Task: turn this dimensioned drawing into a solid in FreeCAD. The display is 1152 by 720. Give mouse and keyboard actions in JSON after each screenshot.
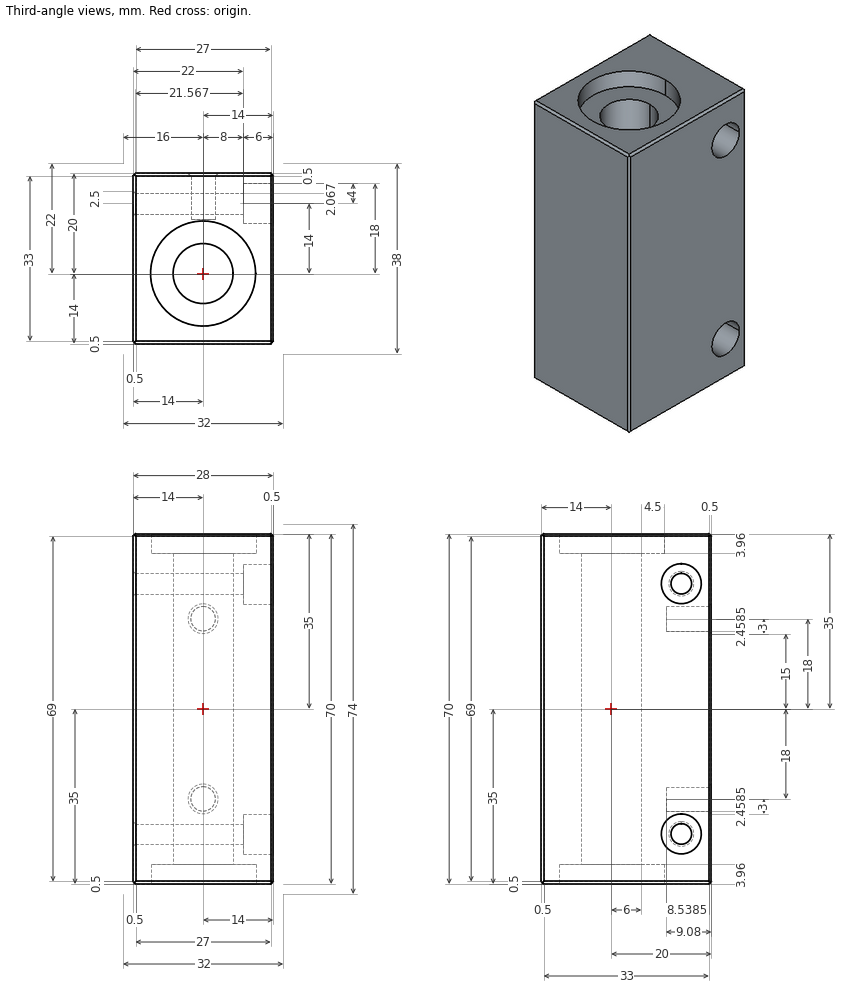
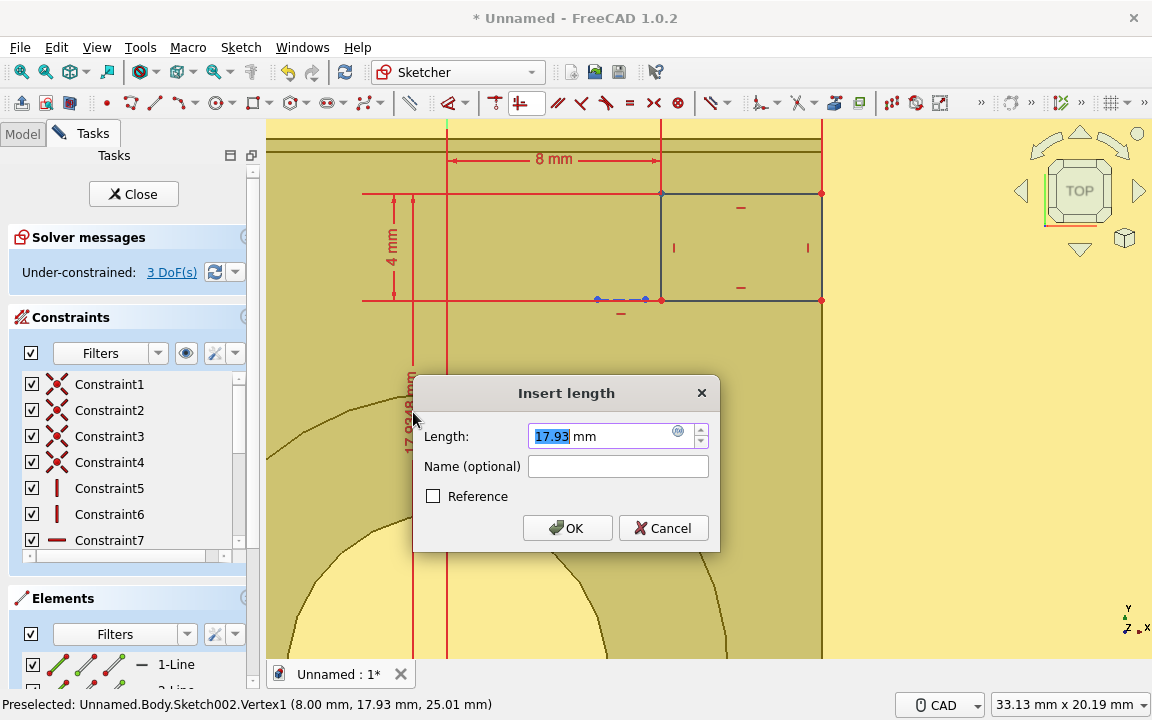
{"action": "type", "text": "18"}
{"action": "key", "text": "Return"}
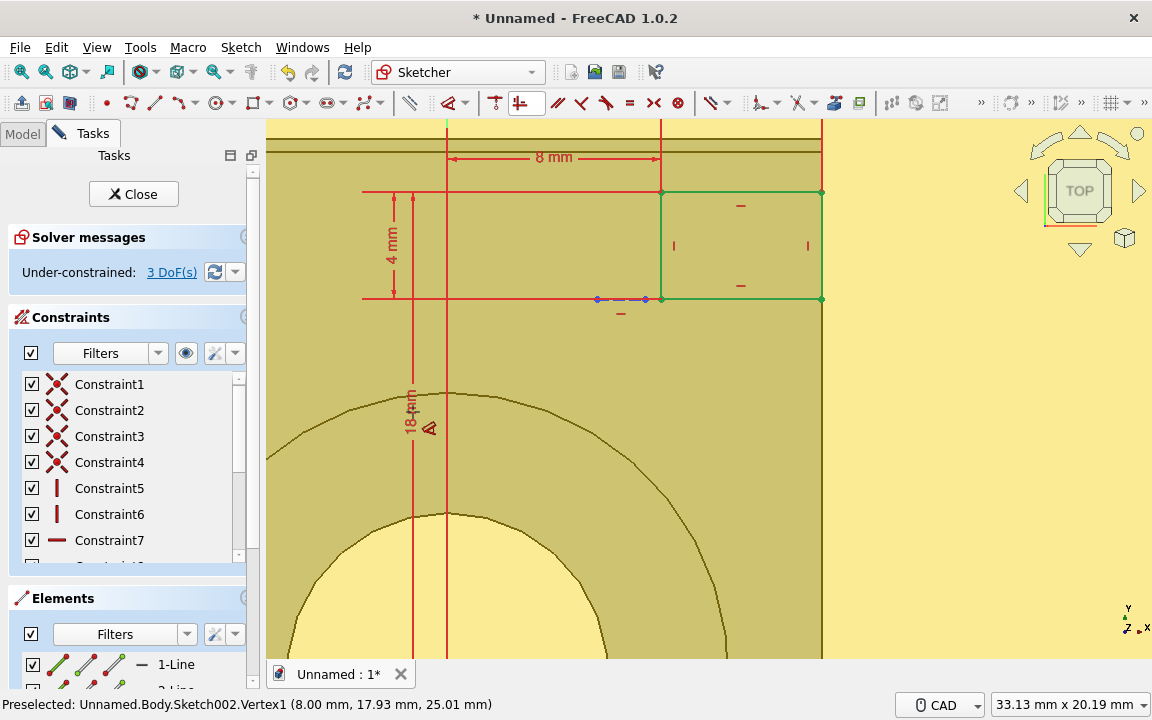
{"action": "left_click", "coordinate": [645, 300]}
{"action": "left_click", "coordinate": [413, 465]}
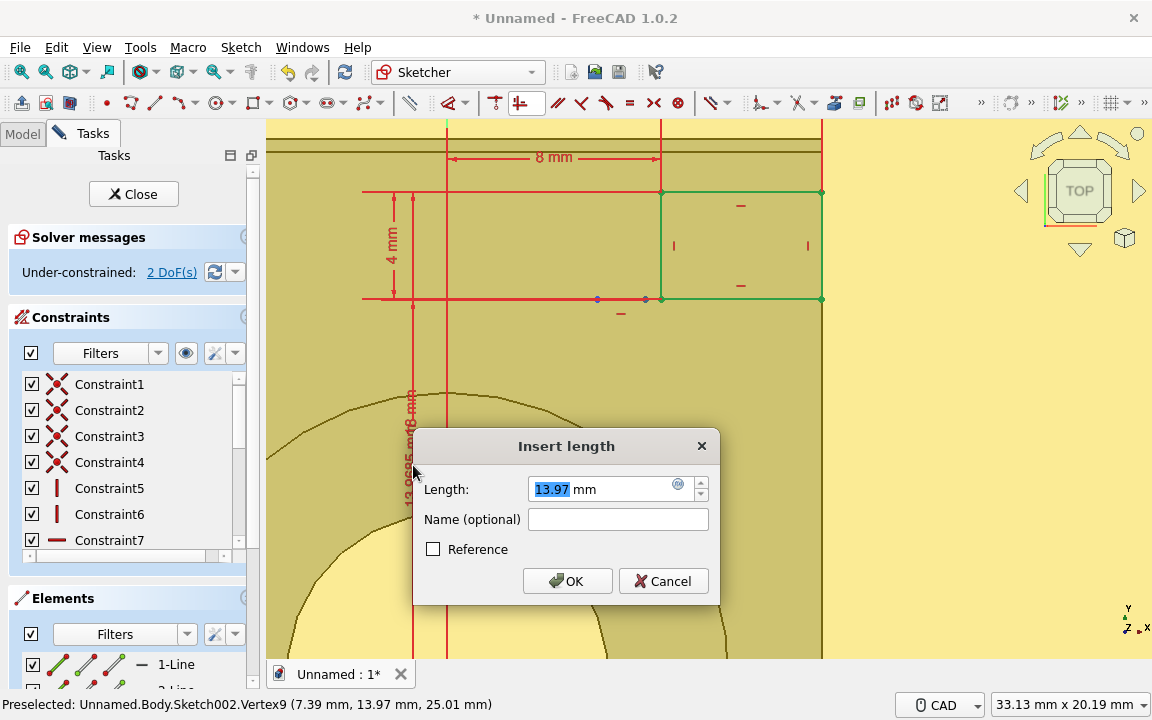
{"action": "type", "text": "14"}
{"action": "key", "text": "Return"}
{"action": "key", "text": "Escape"}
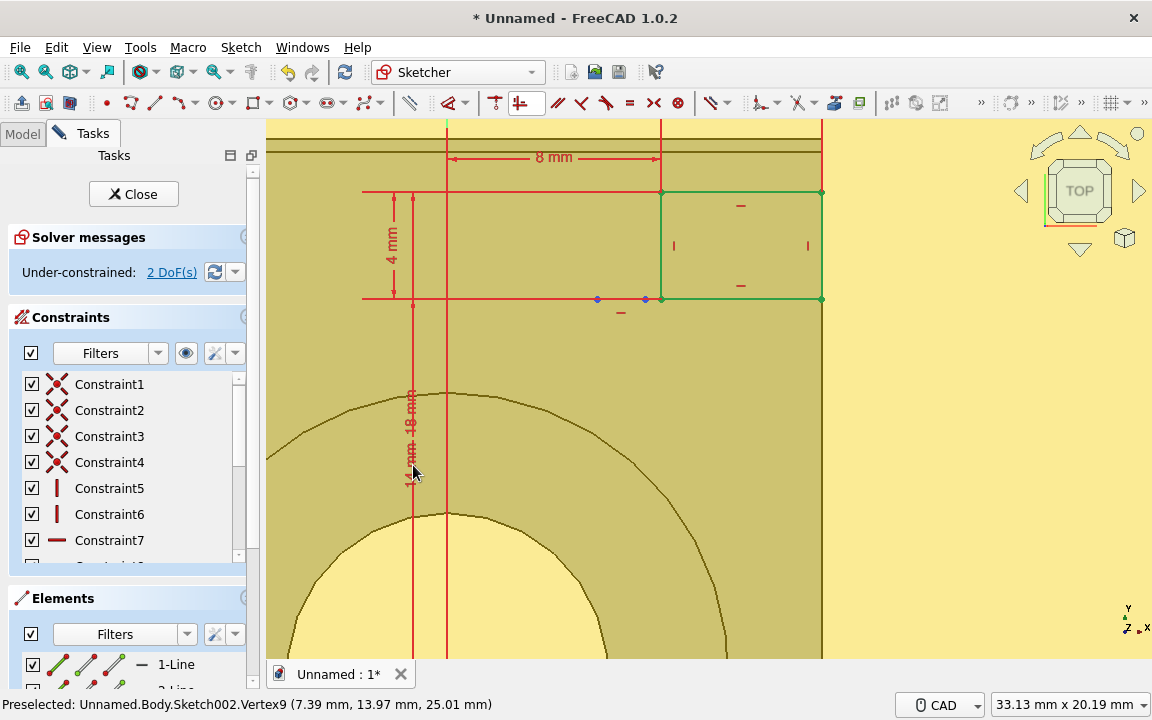
{"action": "left_click", "coordinate": [134, 194]}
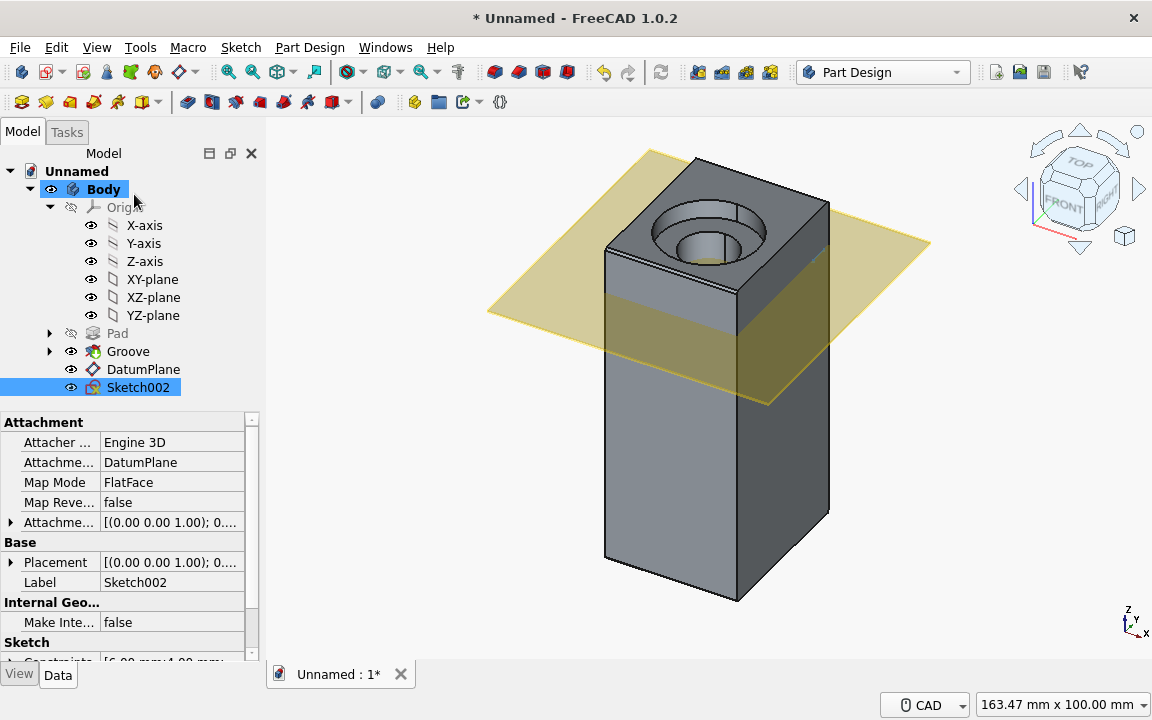
{"action": "left_click", "coordinate": [236, 102]}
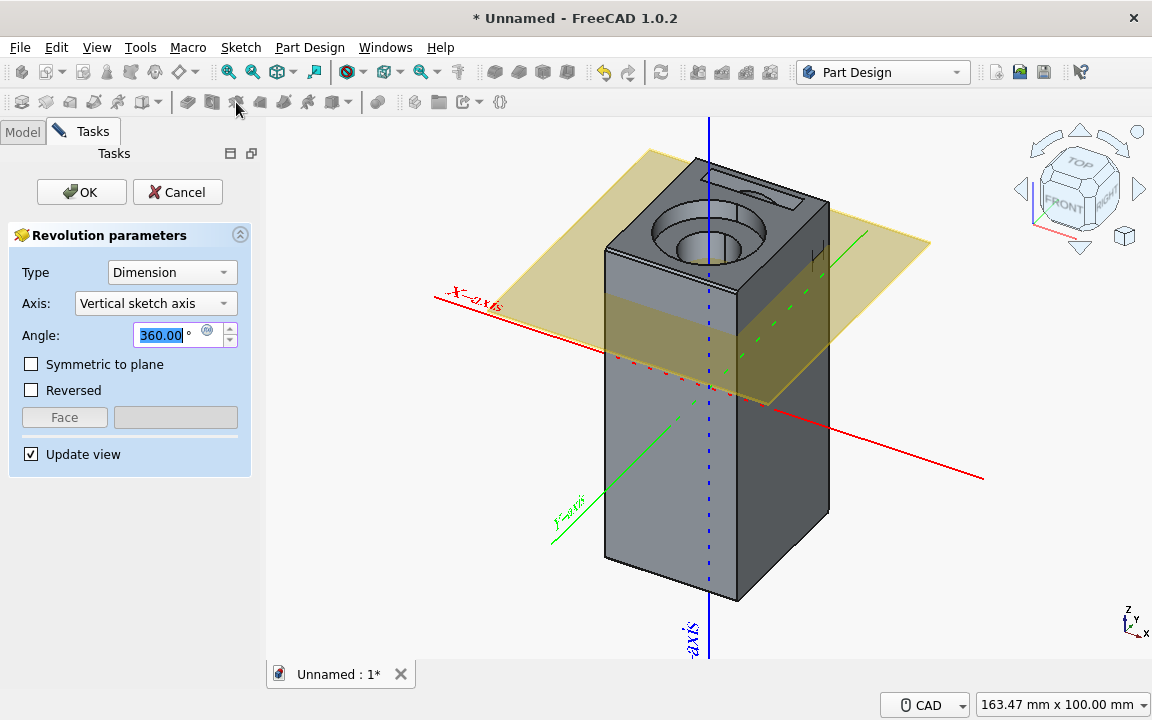
{"action": "left_click", "coordinate": [156, 304]}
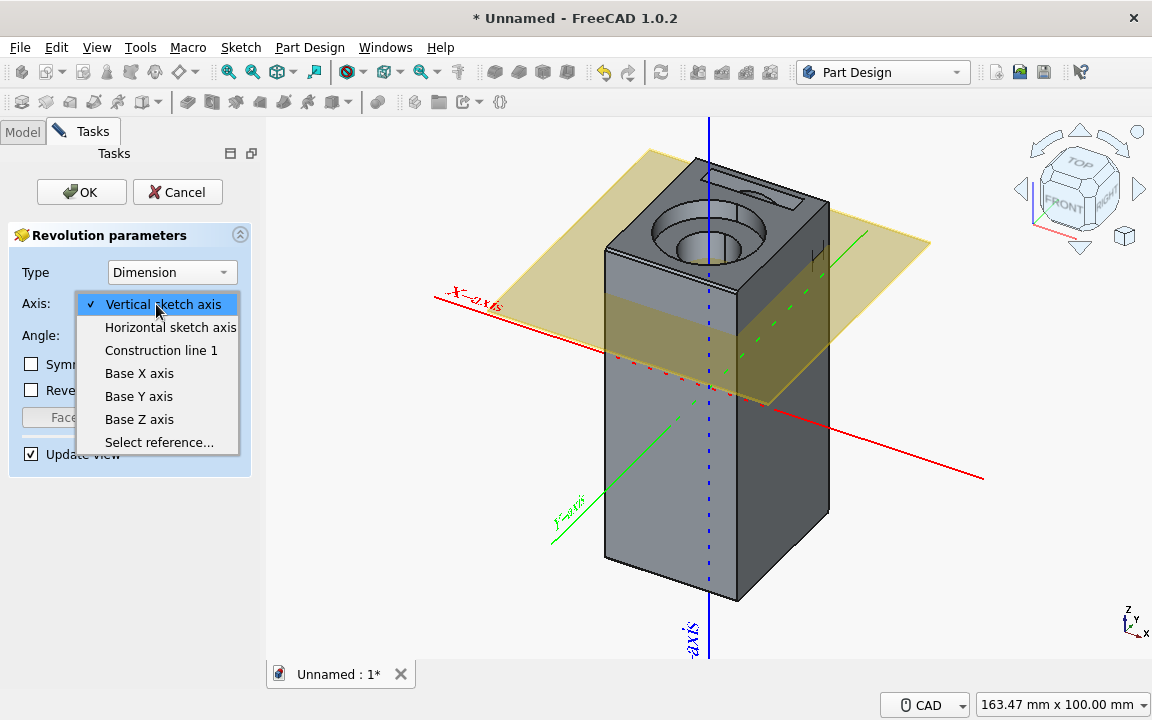
{"action": "left_click", "coordinate": [156, 350]}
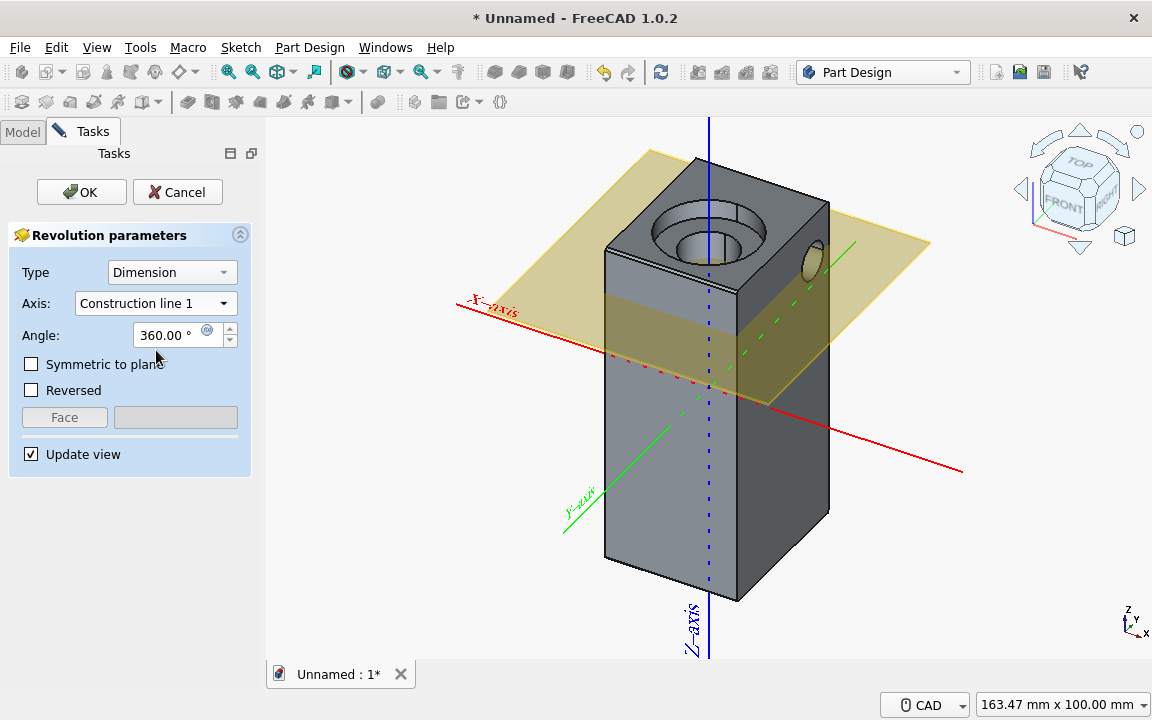
{"action": "left_click", "coordinate": [82, 192]}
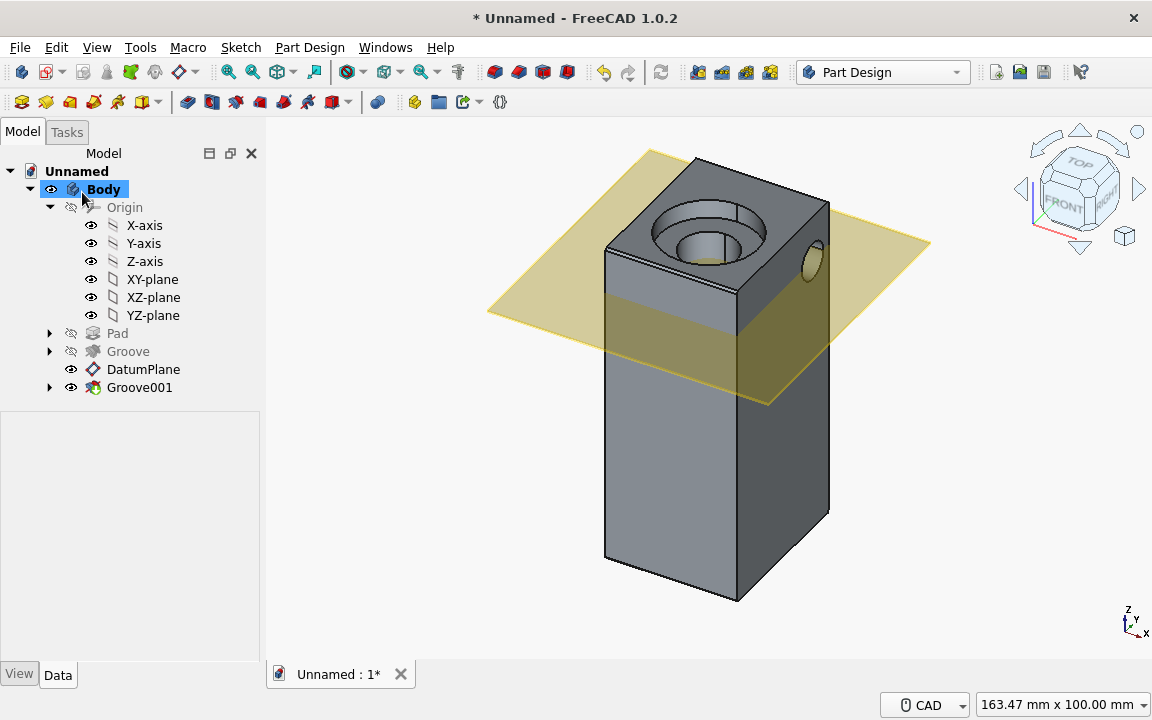
{"action": "left_click", "coordinate": [116, 369]}
{"action": "key", "text": "space"}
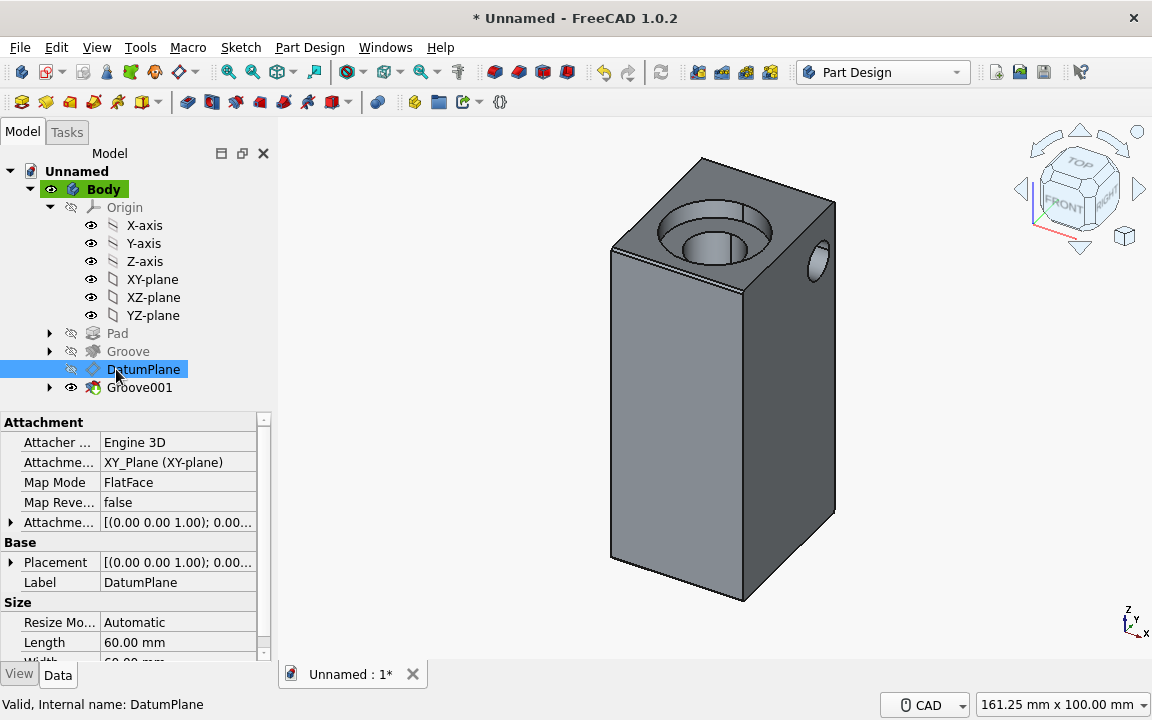
{"action": "left_click", "coordinate": [136, 279]}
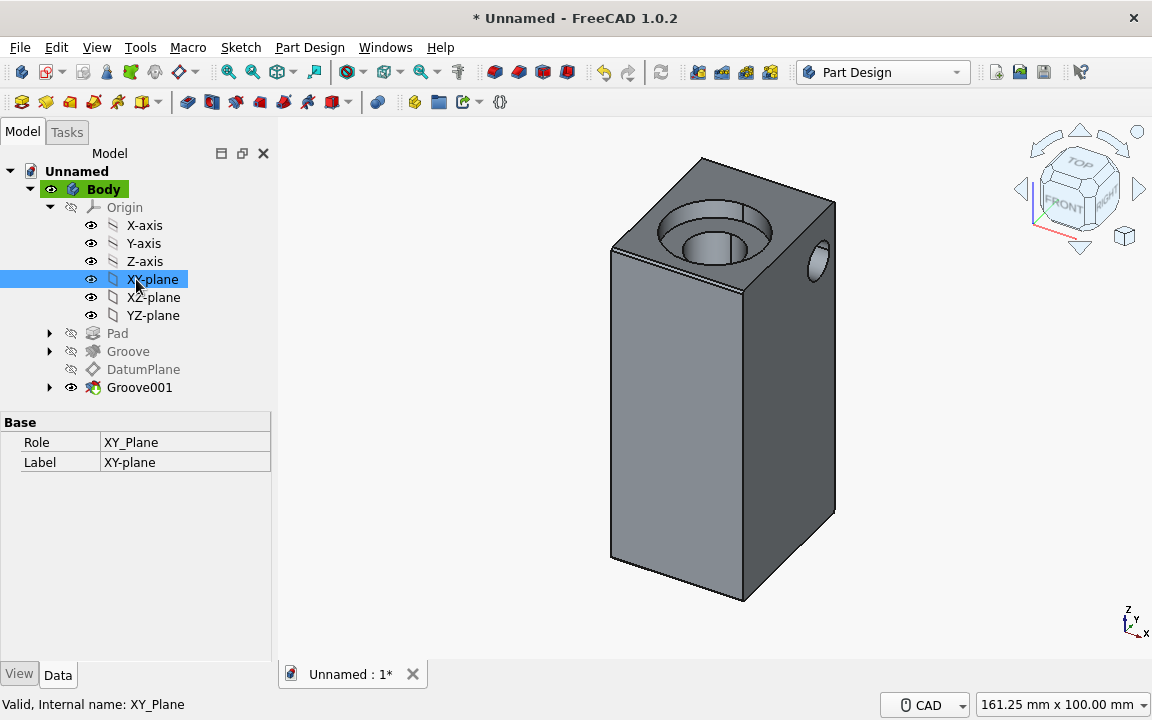
{"action": "left_click", "coordinate": [180, 72]}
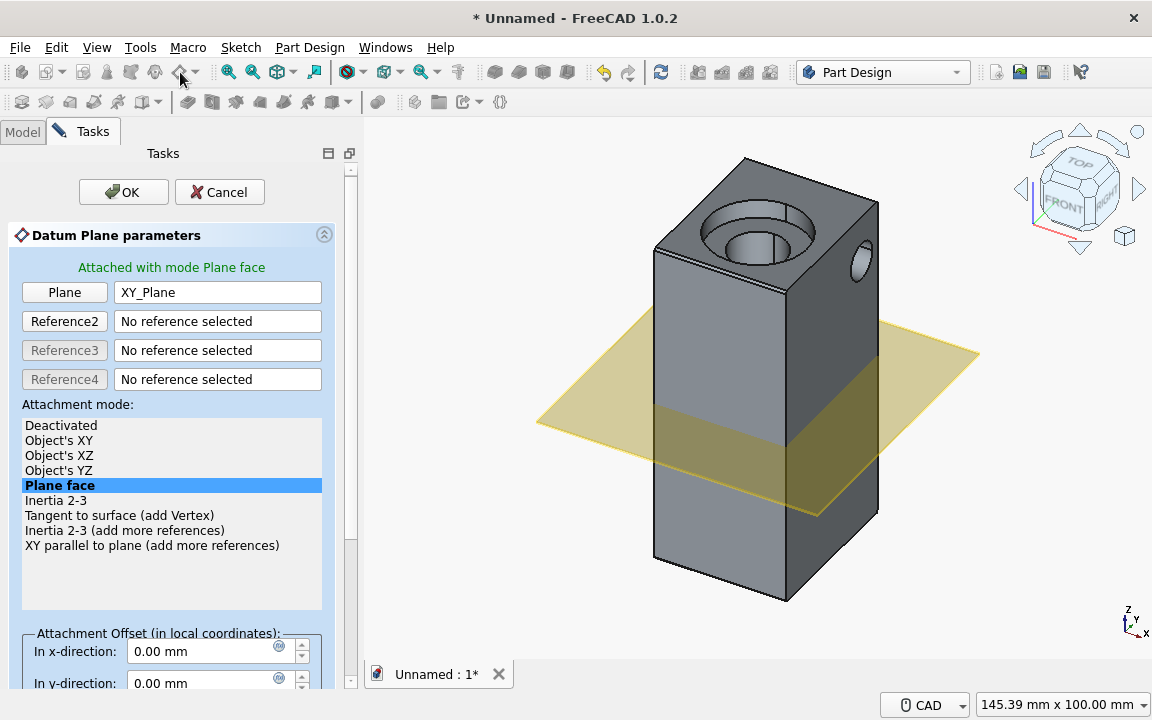
{"action": "scroll", "coordinate": [351, 426], "scroll_direction": "down", "scroll_amount": 2}